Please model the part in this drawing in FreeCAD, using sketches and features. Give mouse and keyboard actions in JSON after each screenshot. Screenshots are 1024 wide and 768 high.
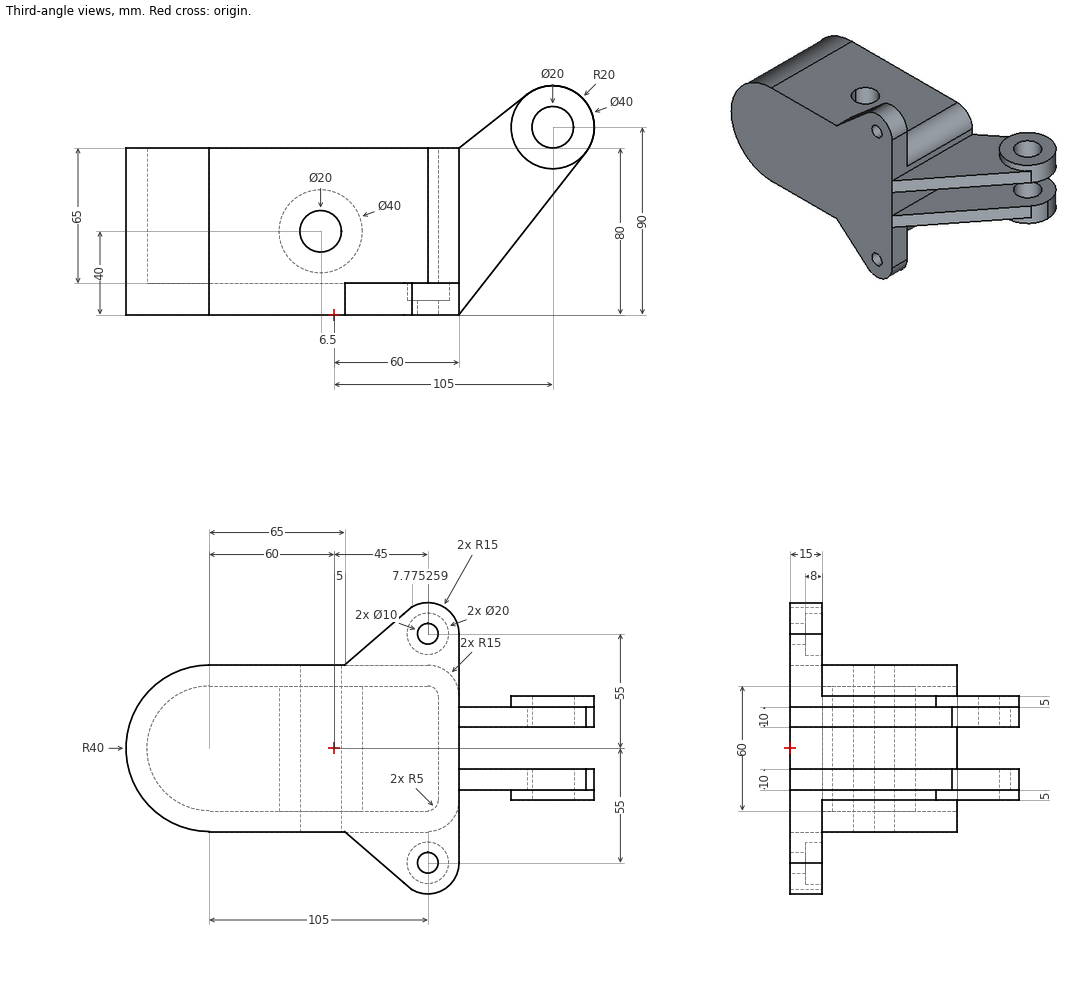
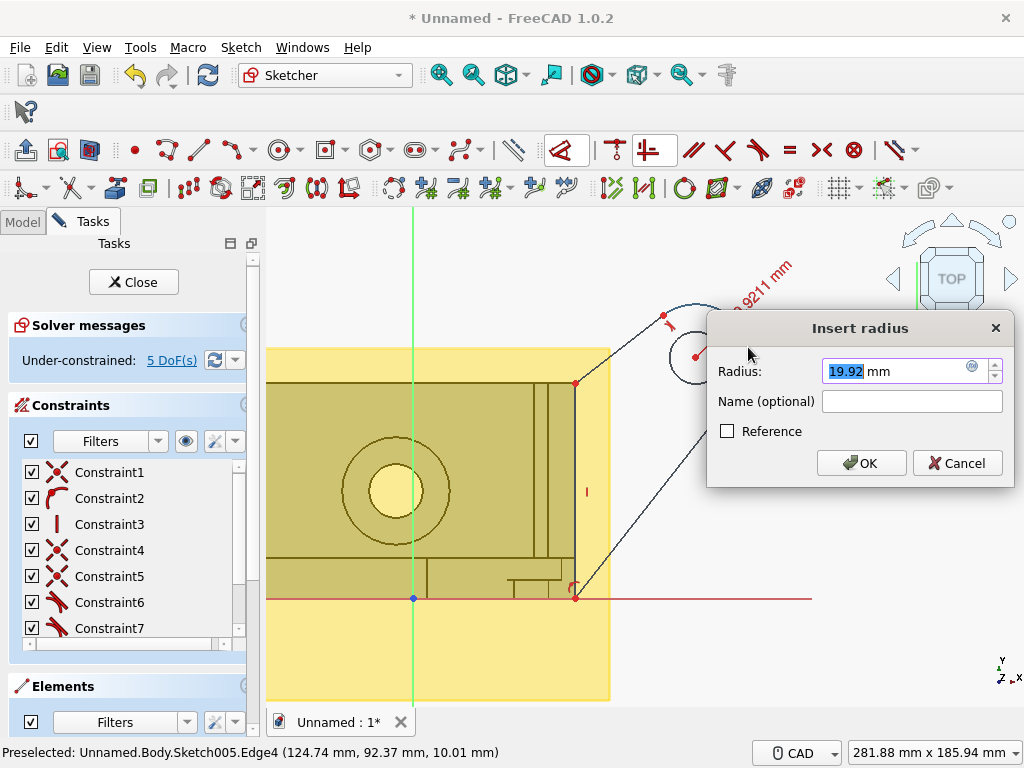
{"action": "type", "text": "20"}
{"action": "key", "text": "Return"}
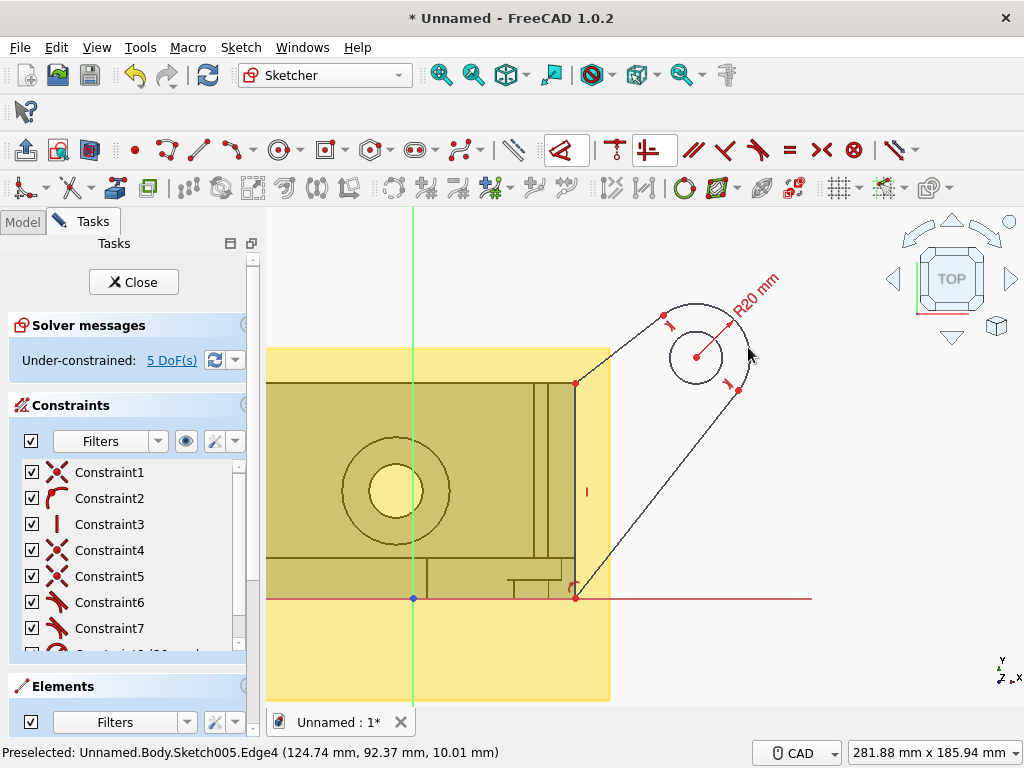
{"action": "left_click", "coordinate": [715, 339]}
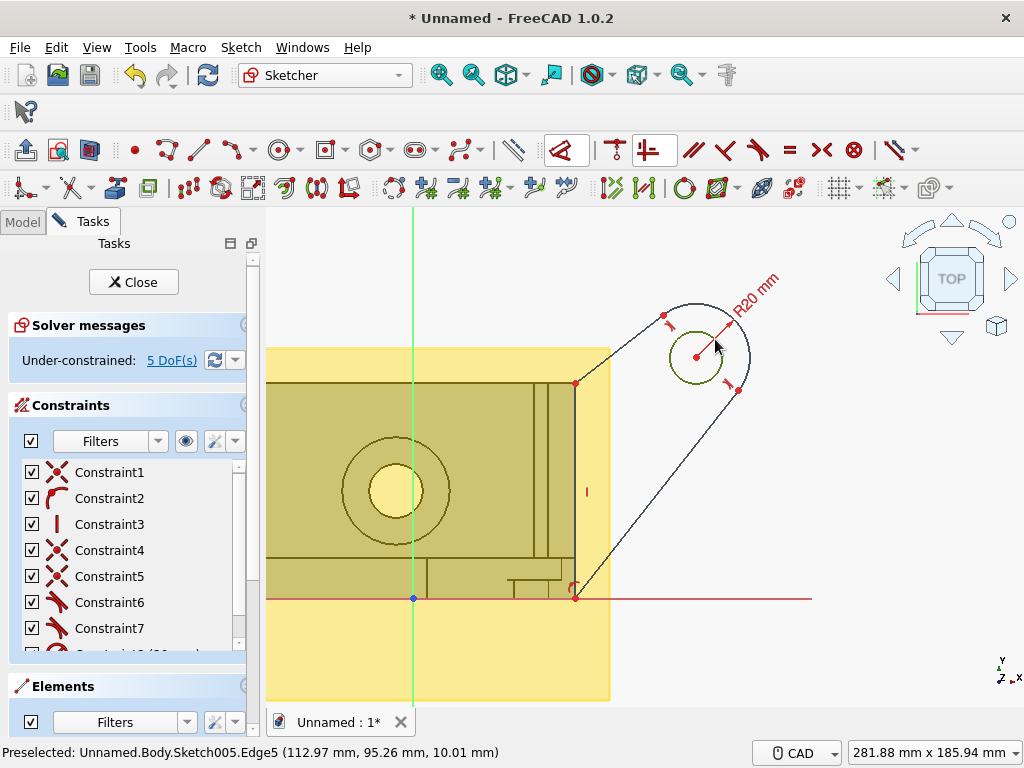
{"action": "left_click", "coordinate": [584, 150]}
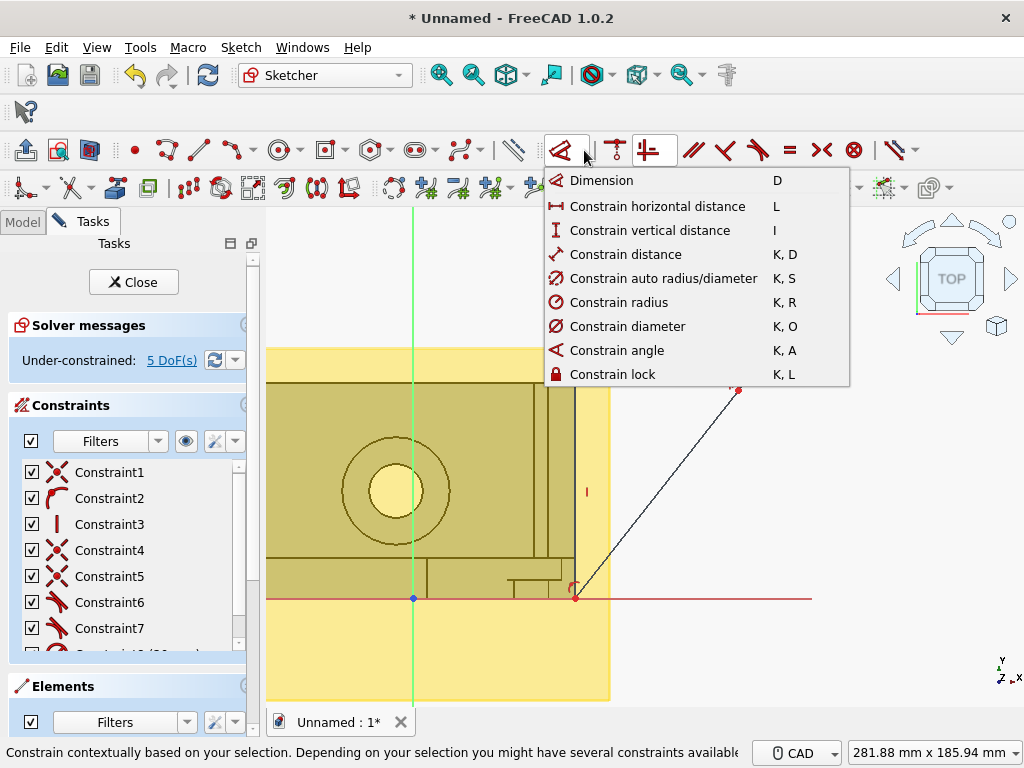
{"action": "left_click", "coordinate": [697, 326]}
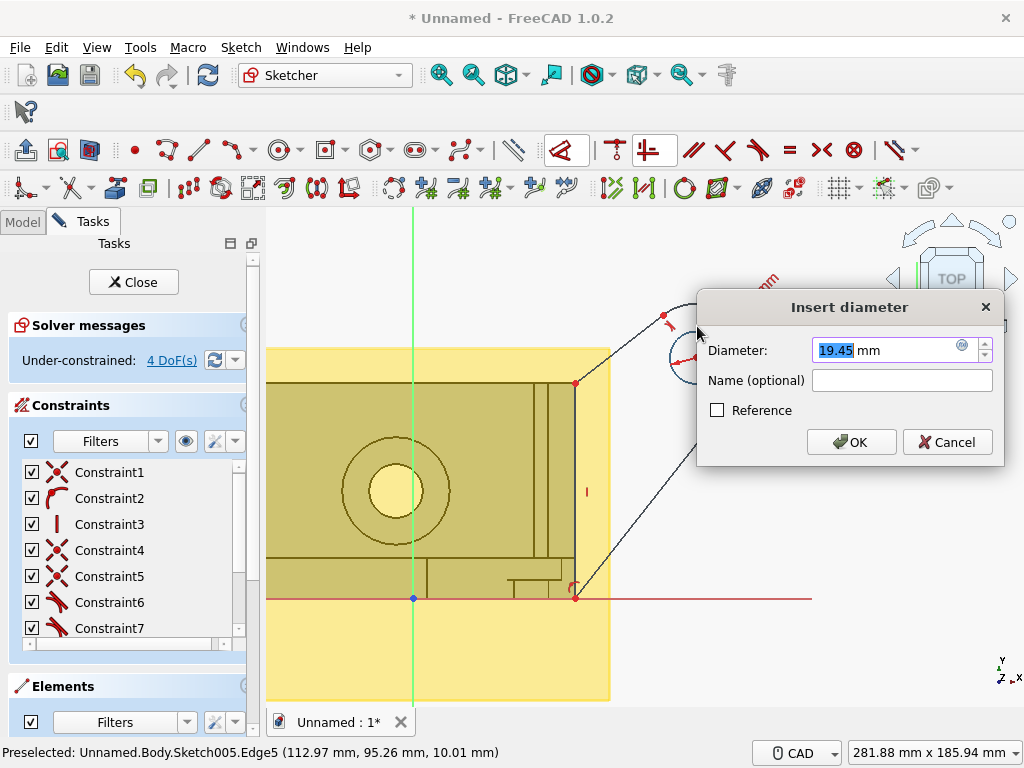
{"action": "type", "text": "20"}
{"action": "key", "text": "Return"}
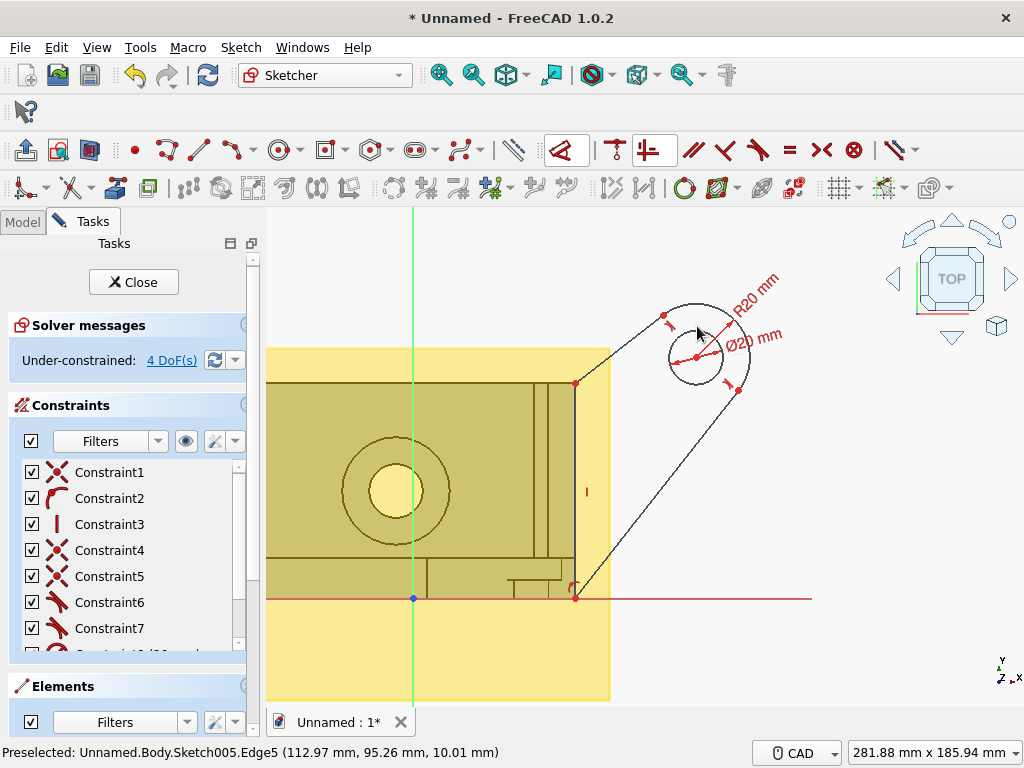
{"action": "left_click", "coordinate": [575, 448]}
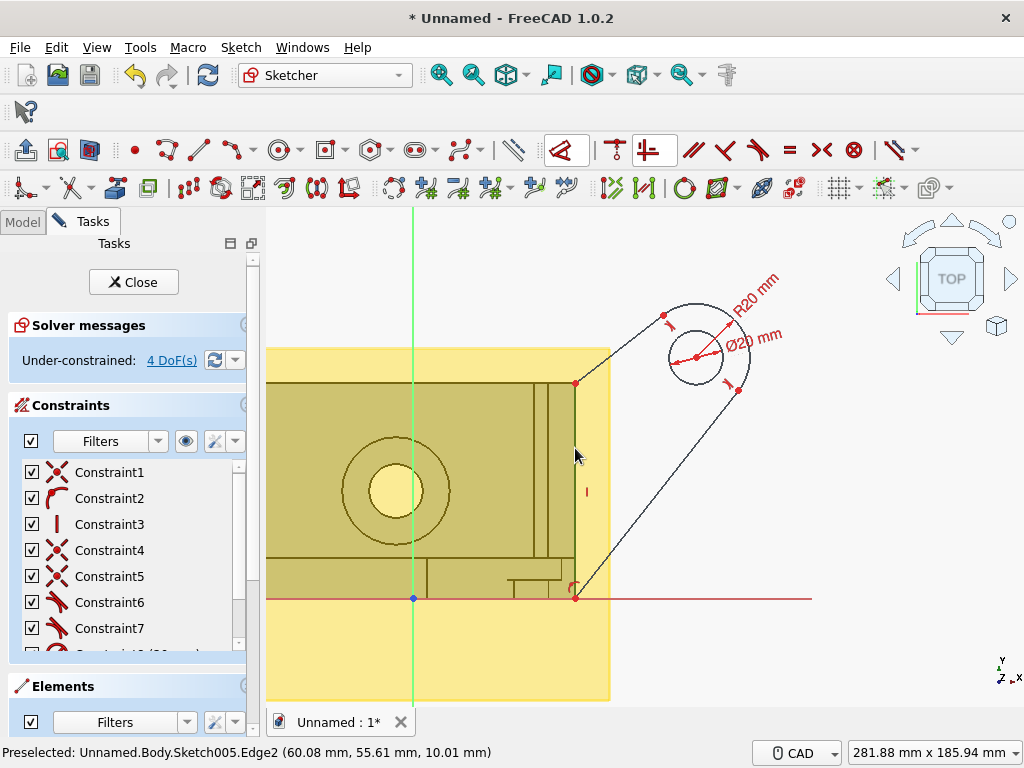
{"action": "key", "text": "i"}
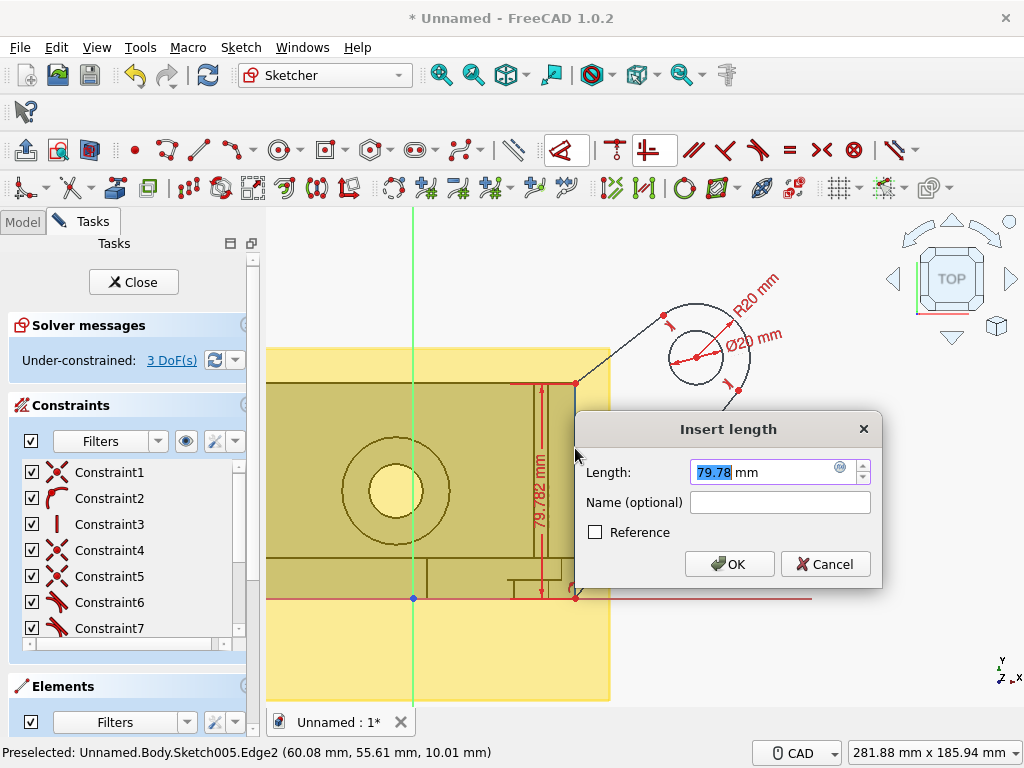
{"action": "type", "text": "80"}
{"action": "key", "text": "Return"}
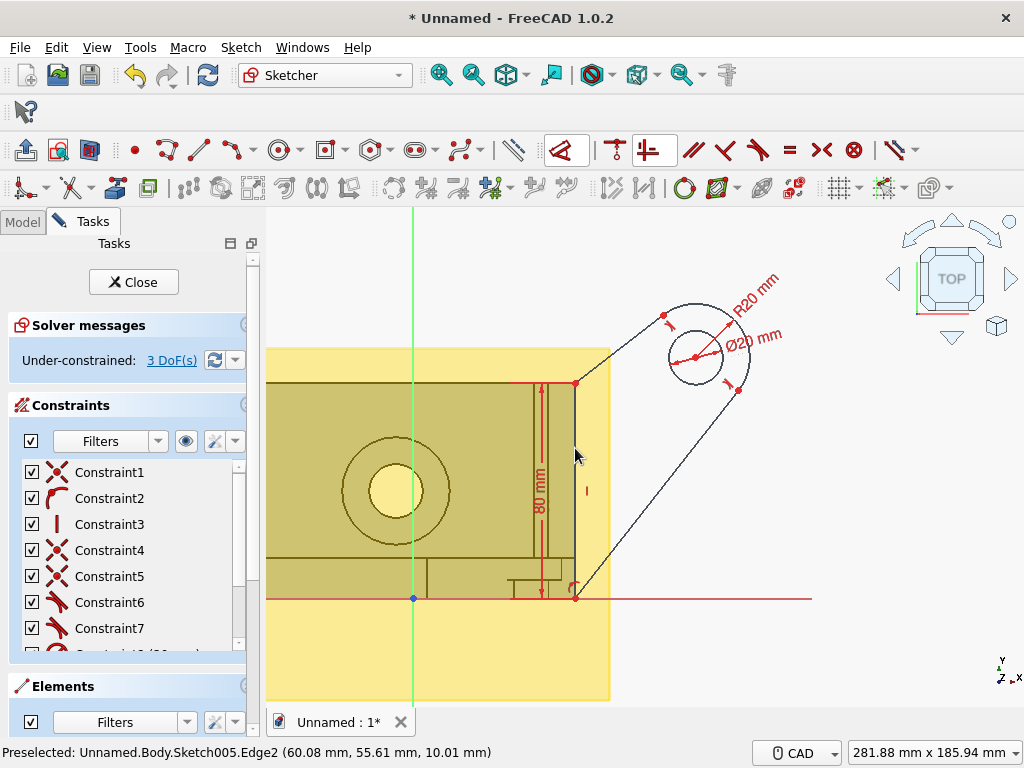
{"action": "left_click", "coordinate": [696, 358]}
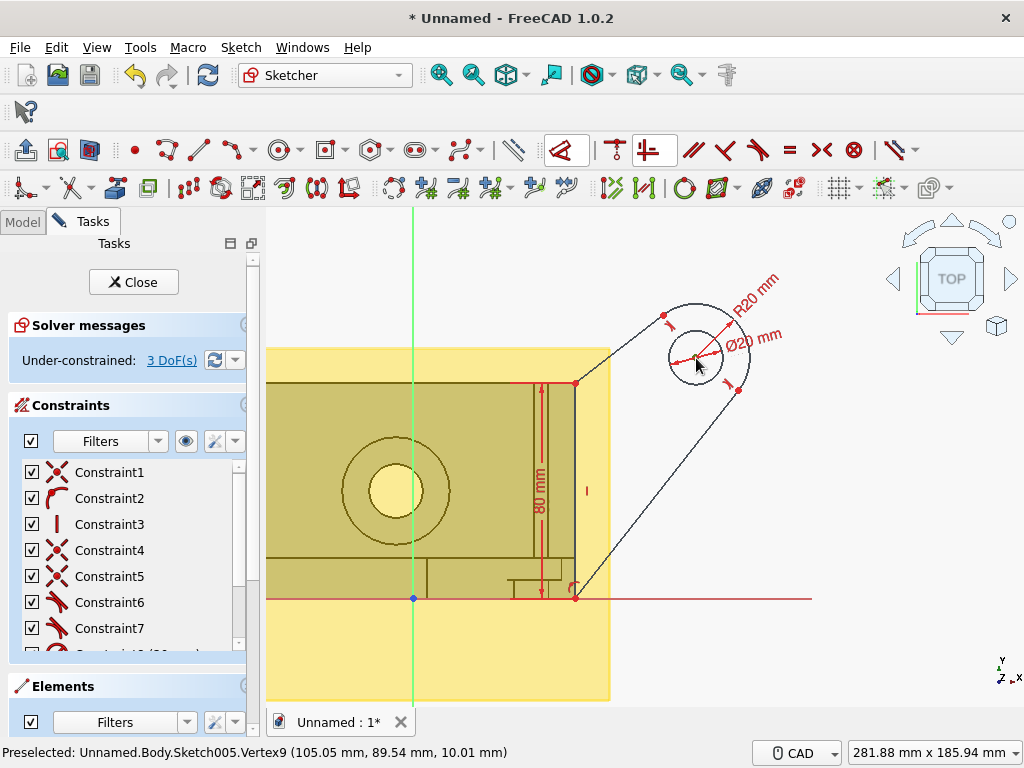
{"action": "key", "text": "i"}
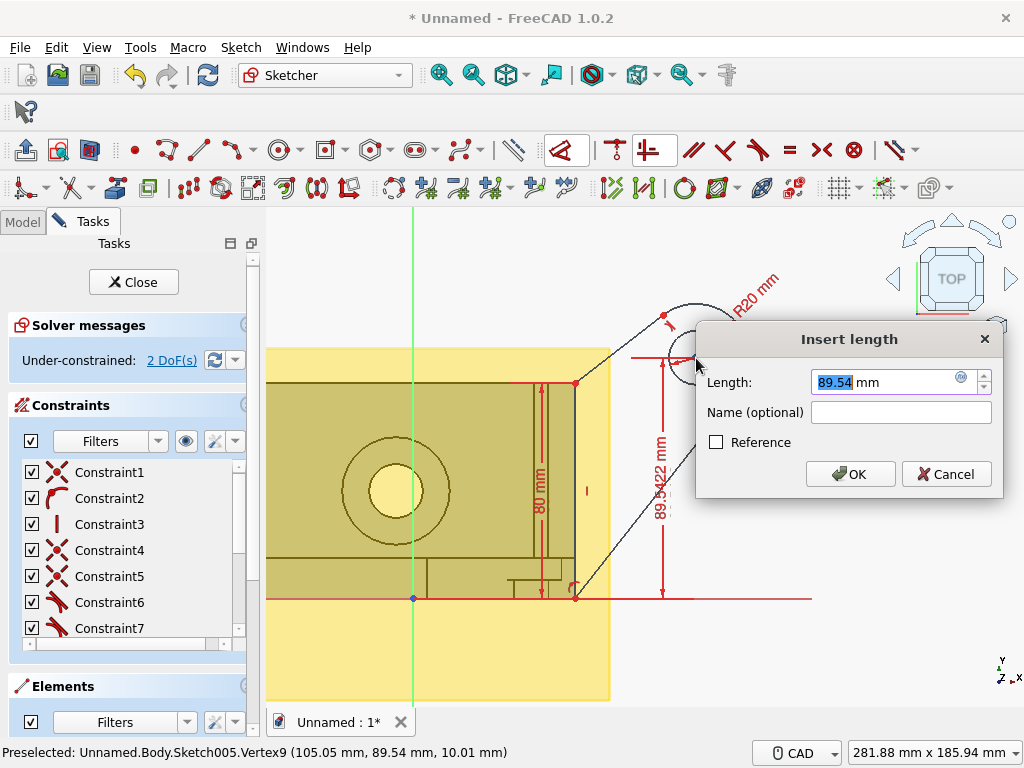
{"action": "type", "text": "90"}
{"action": "key", "text": "Return"}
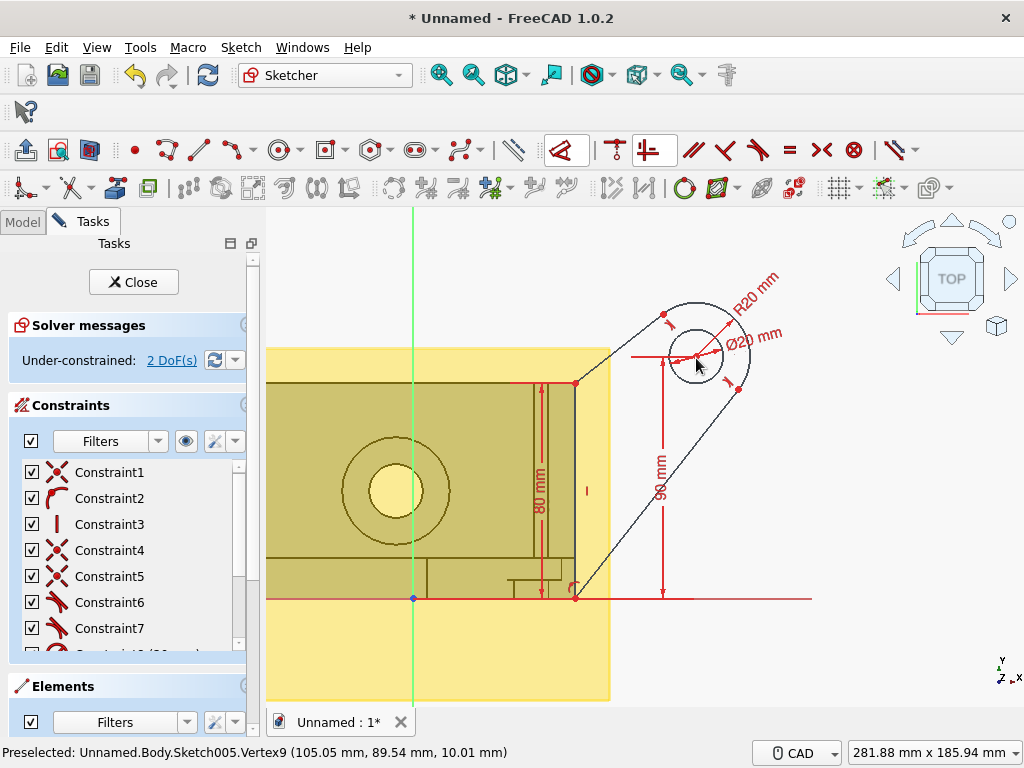
{"action": "left_click", "coordinate": [575, 383]}